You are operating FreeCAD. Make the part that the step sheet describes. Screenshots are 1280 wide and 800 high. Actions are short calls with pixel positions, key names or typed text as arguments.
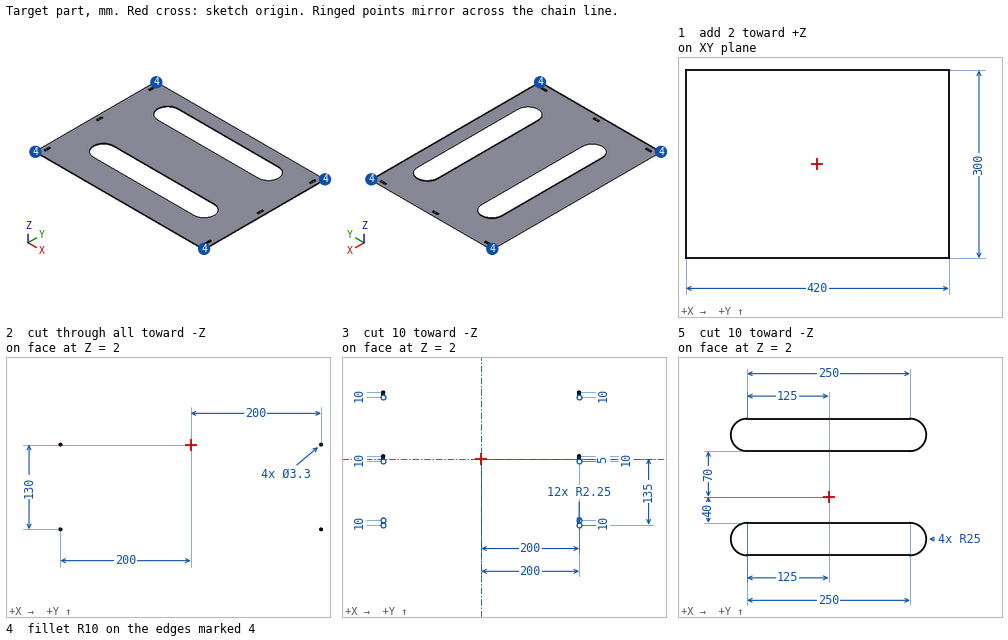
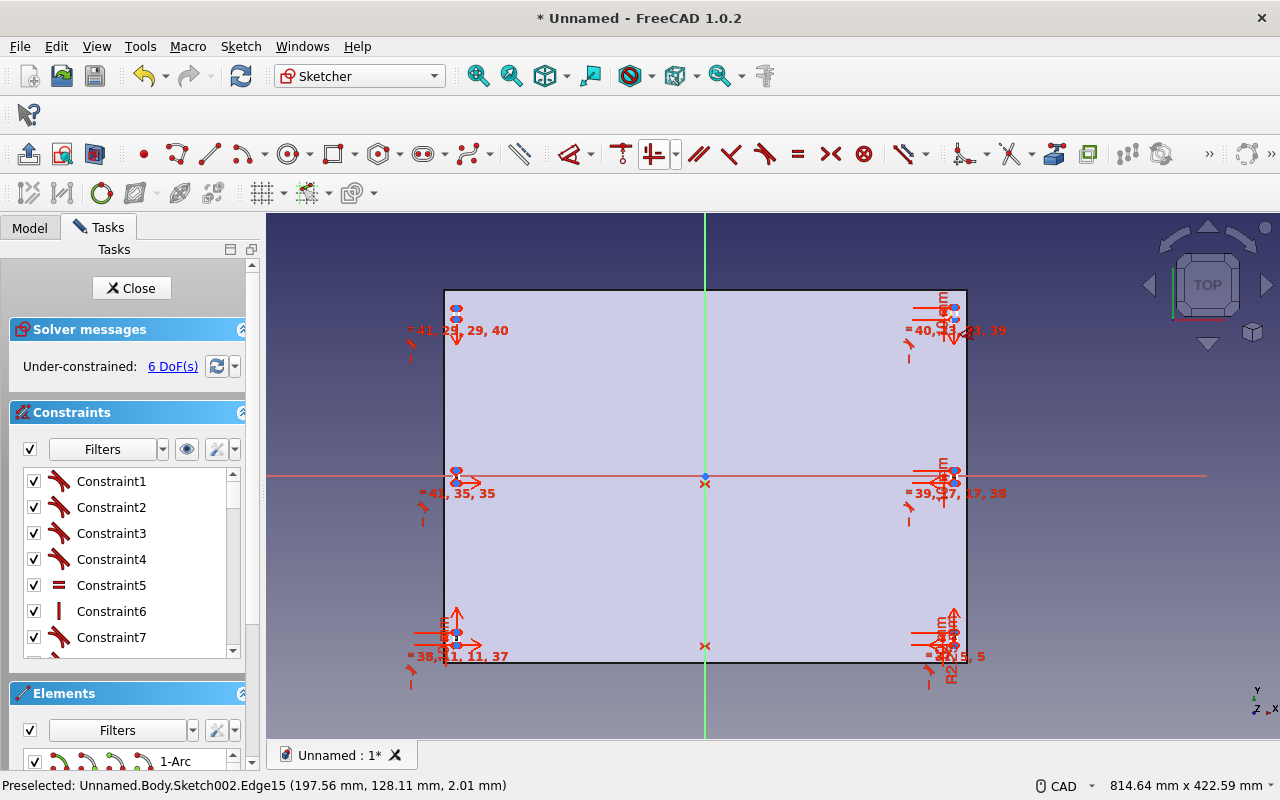
scroll(454, 317, up, 8)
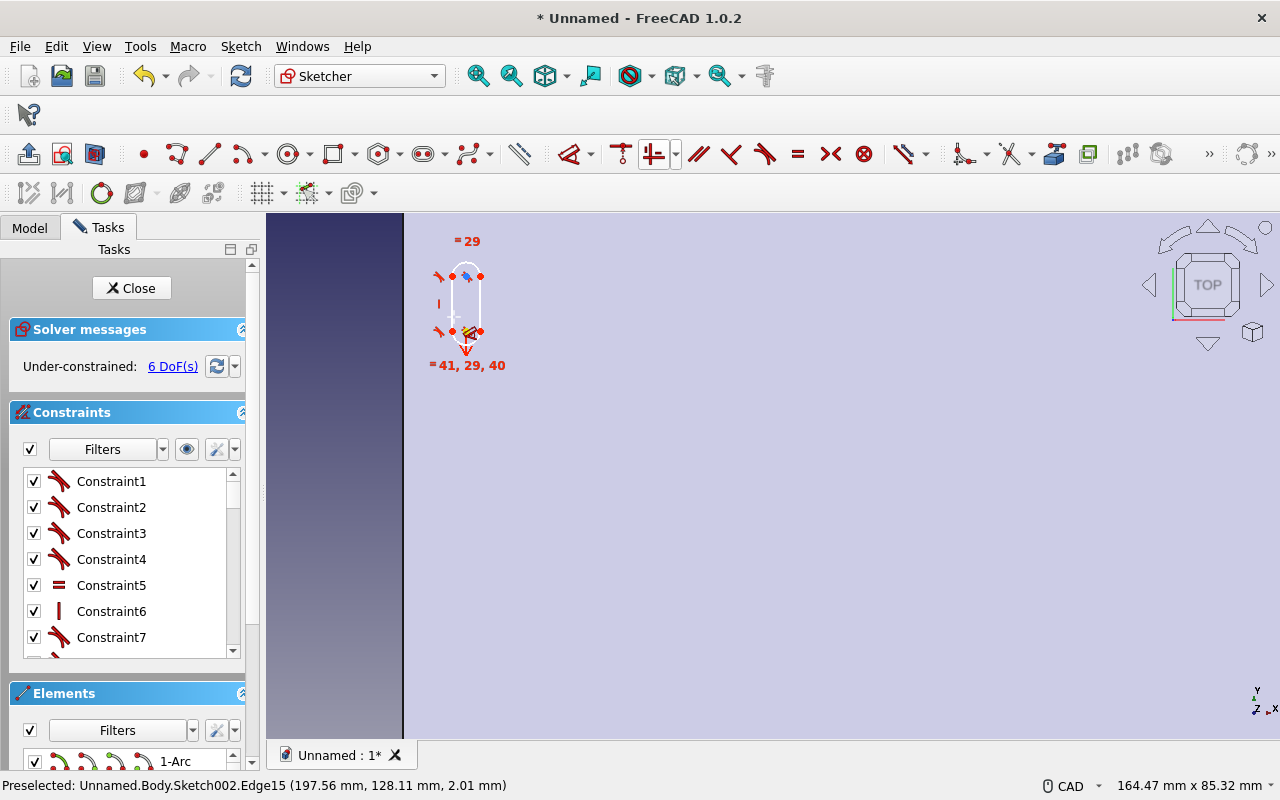
click(452, 315)
click(418, 304)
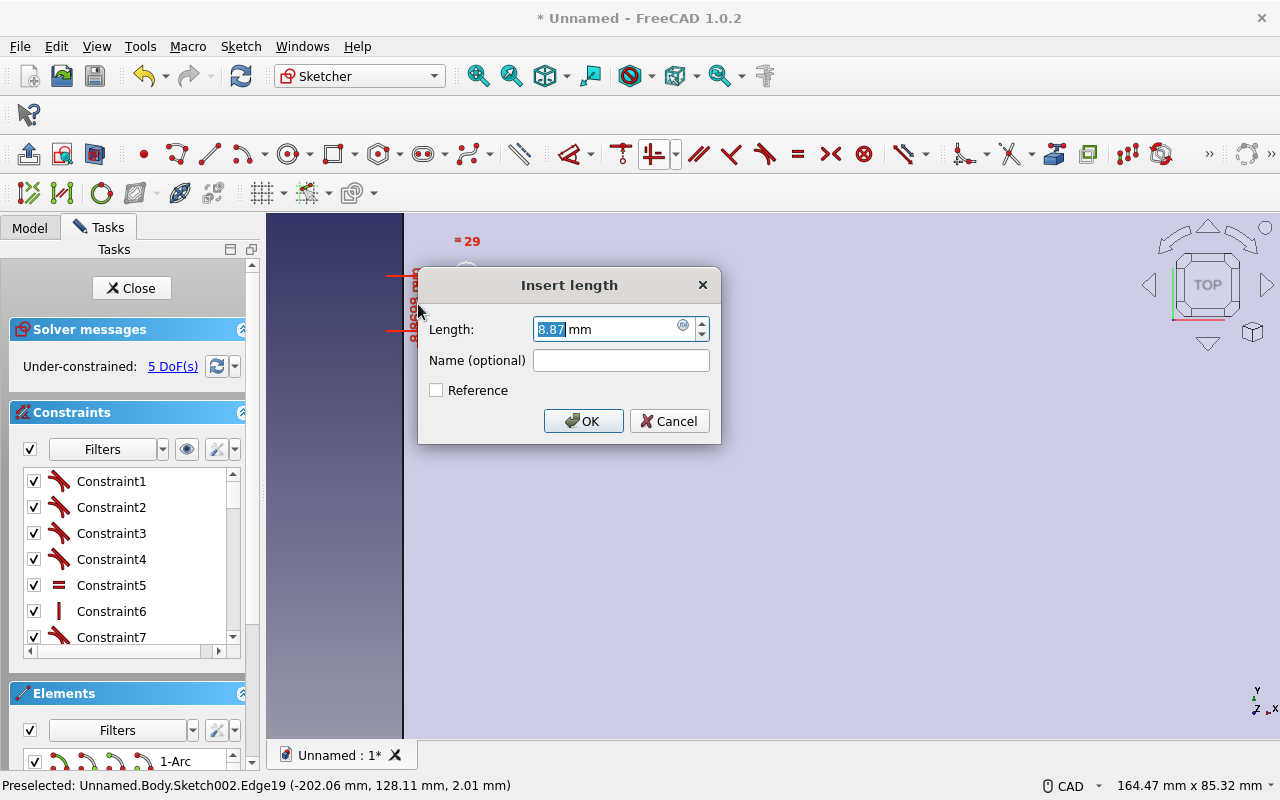
text(10)
key(Return)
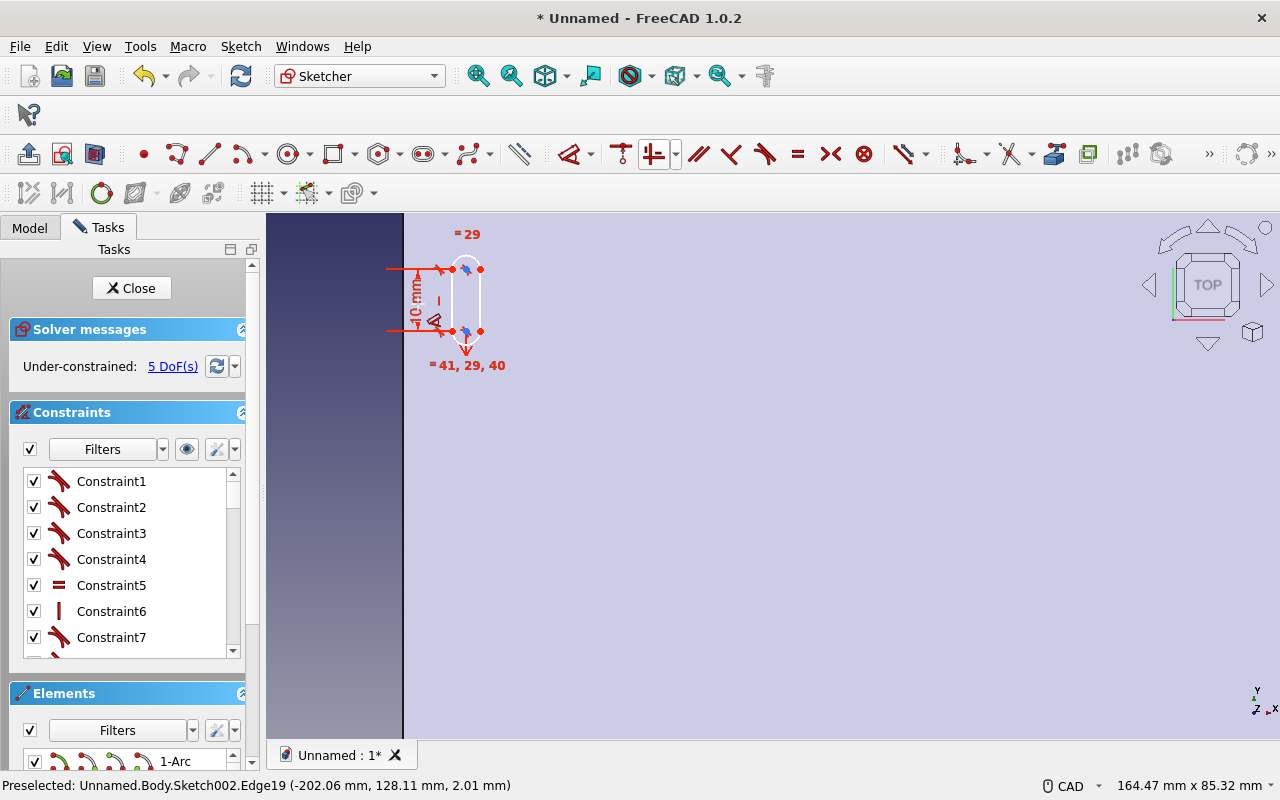
scroll(453, 317, down, 8)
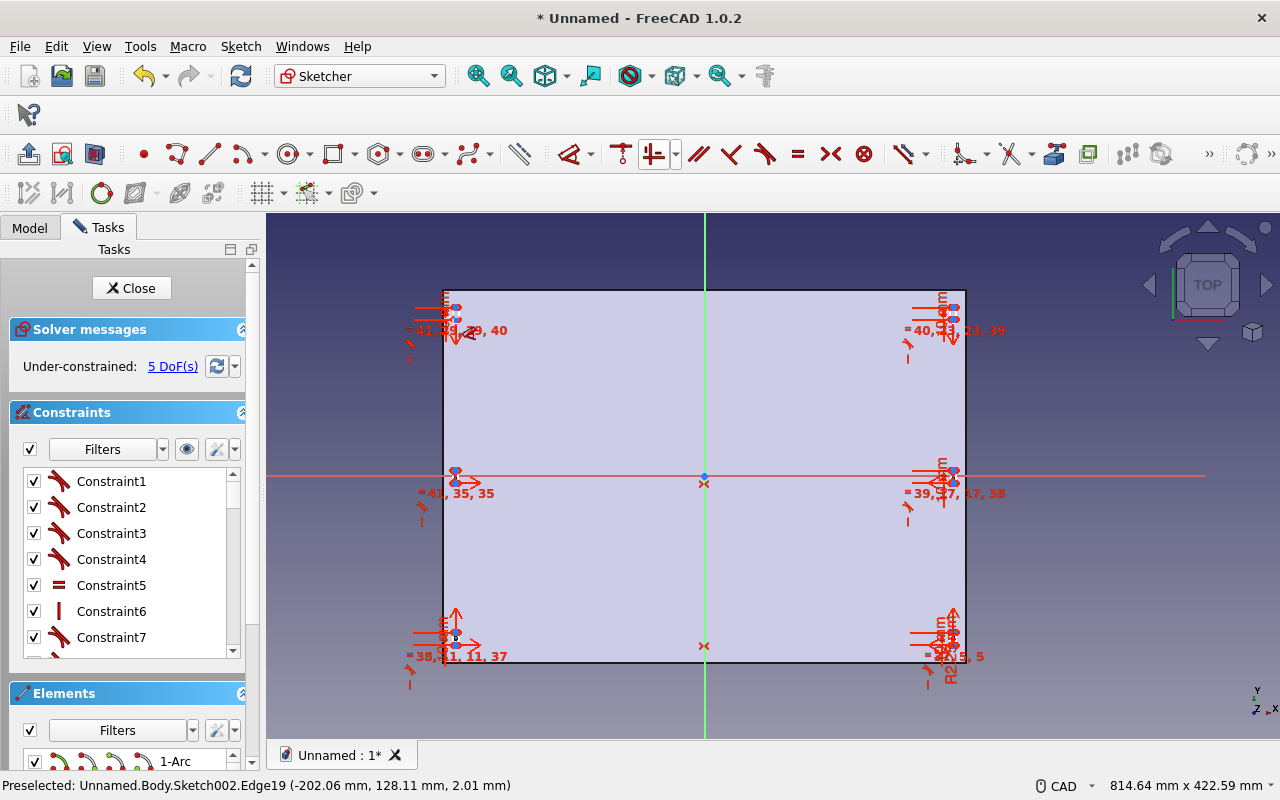
scroll(453, 479, up, 8)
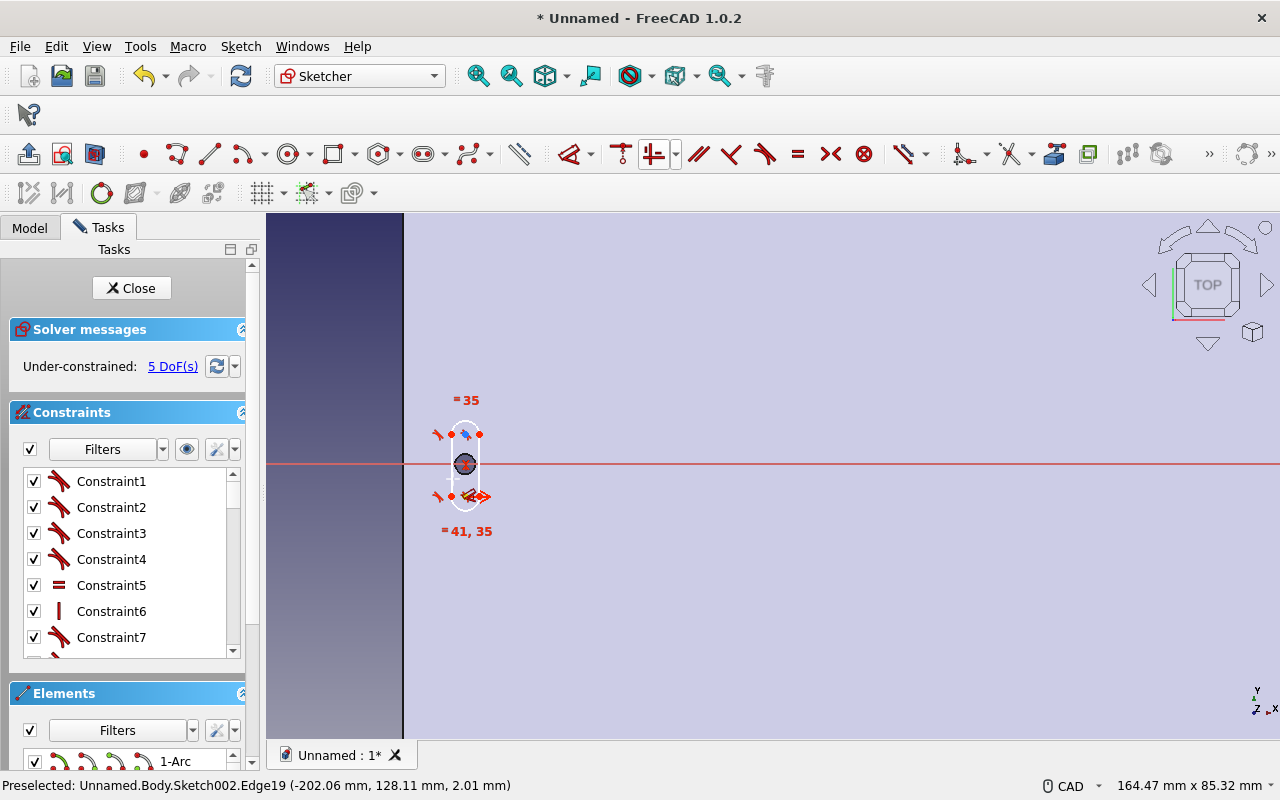
click(452, 478)
click(418, 480)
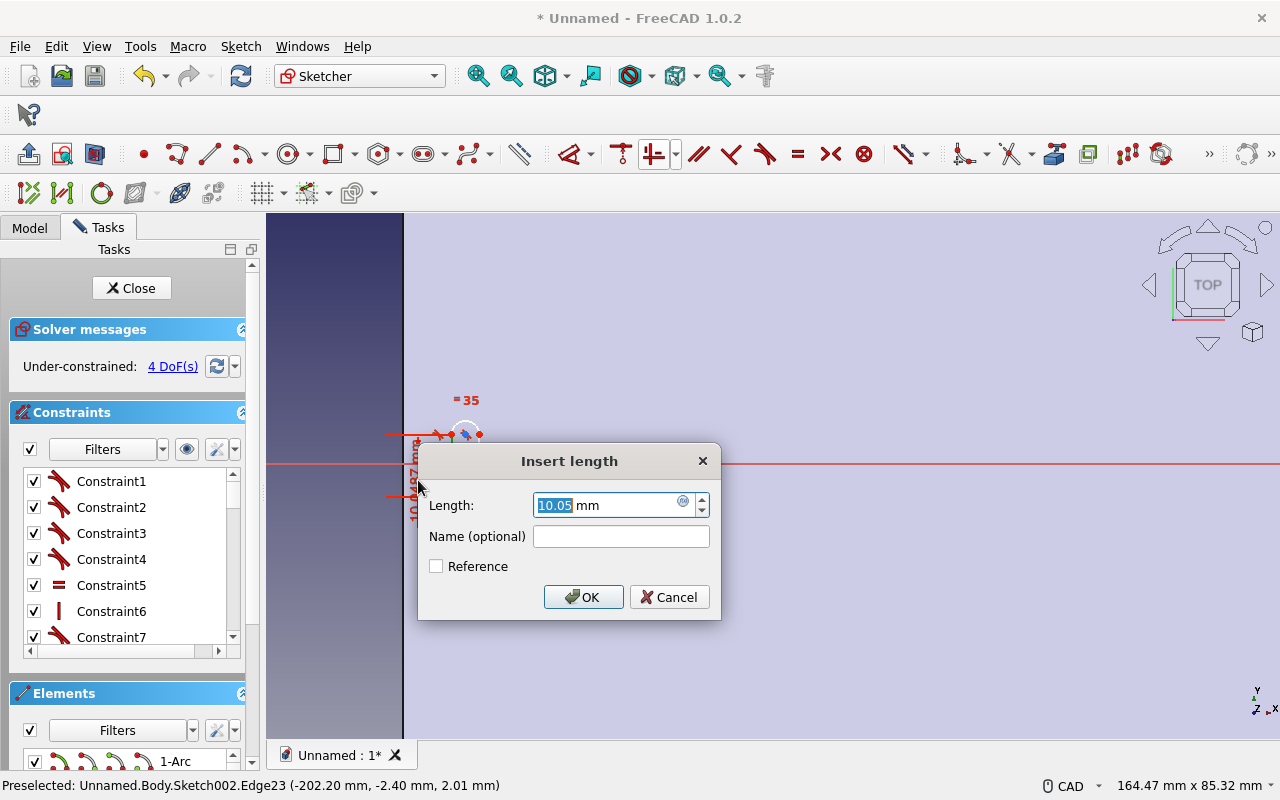
text(10)
key(Return)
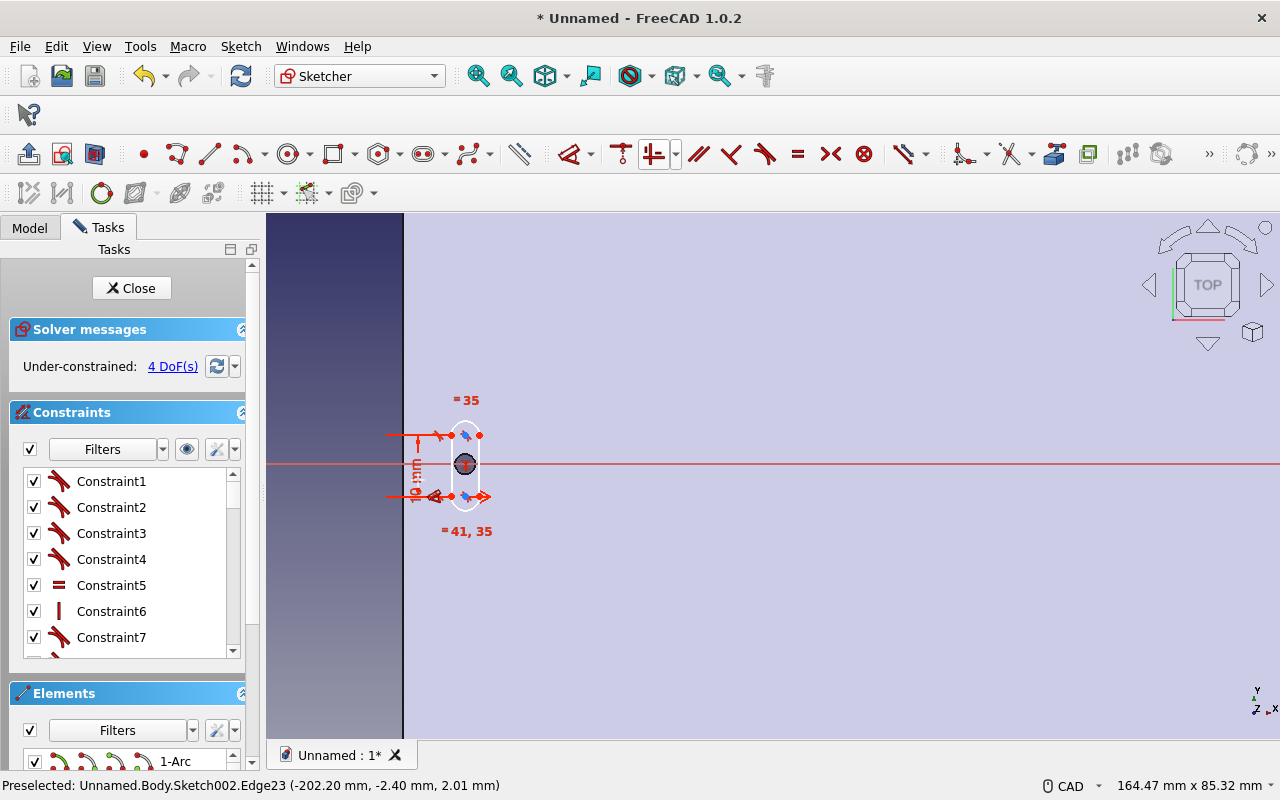
scroll(453, 479, down, 8)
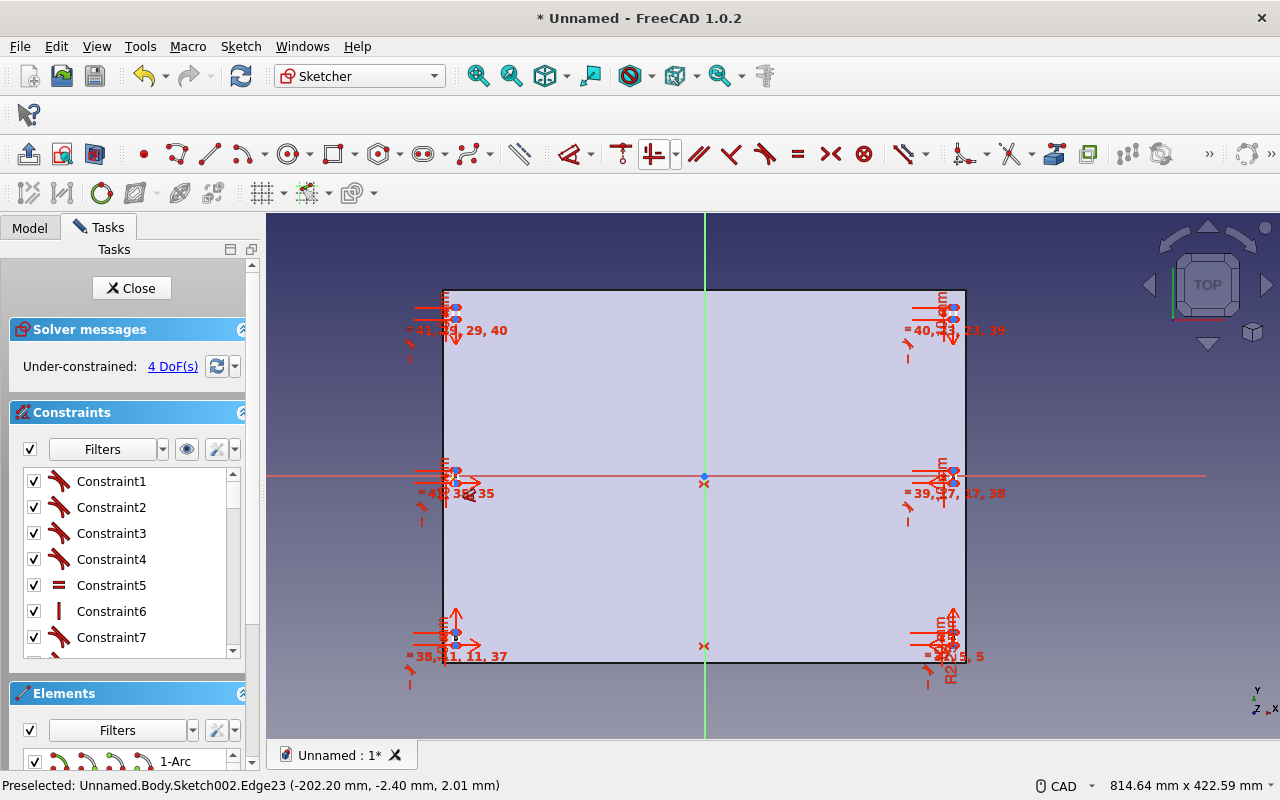
scroll(951, 483, up, 10)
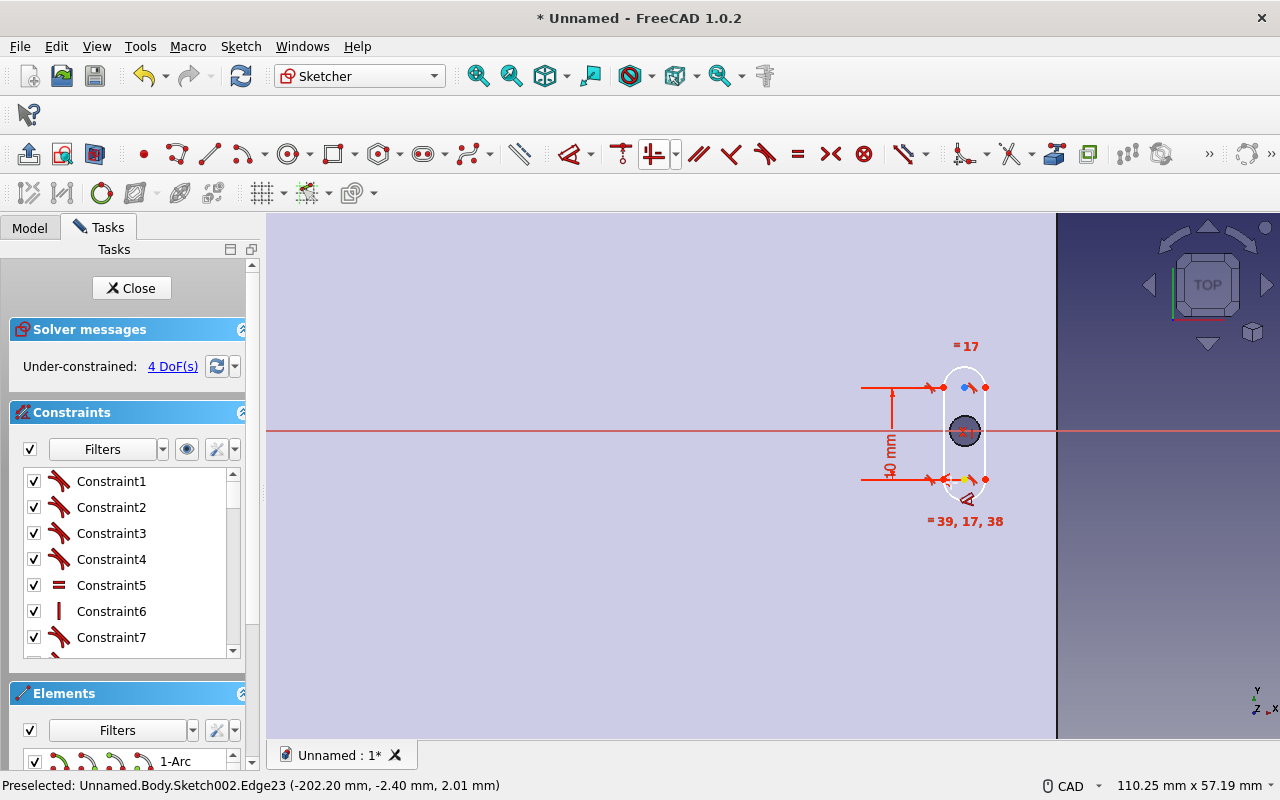
click(944, 480)
click(1002, 455)